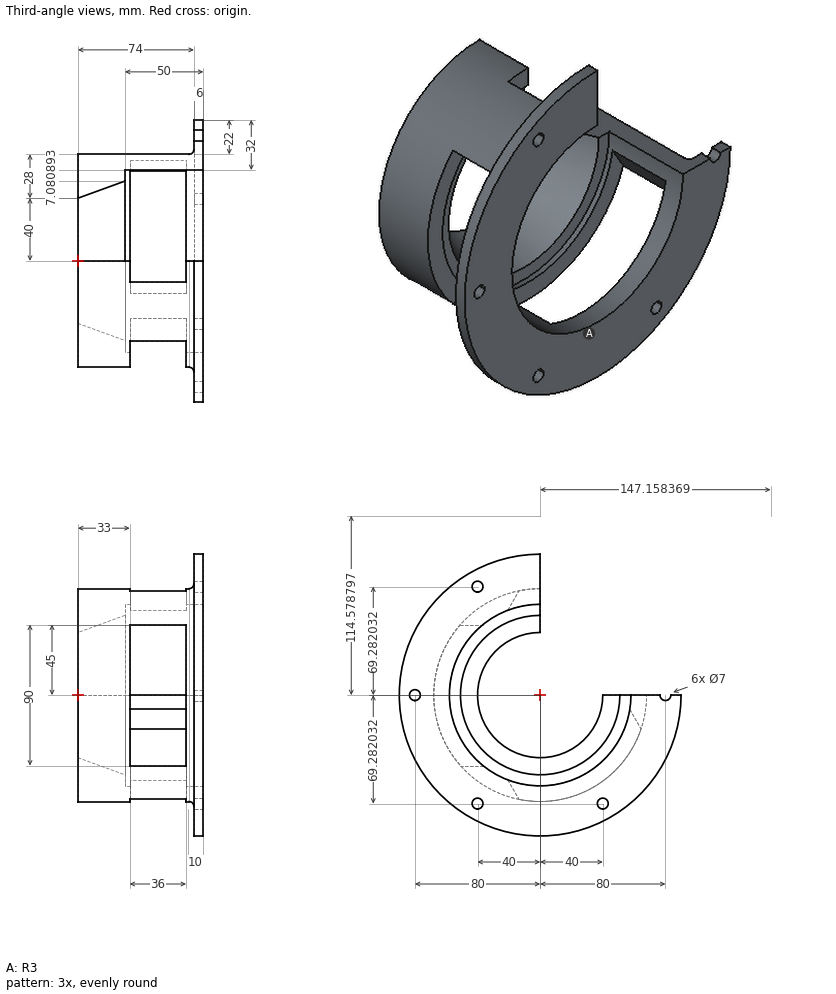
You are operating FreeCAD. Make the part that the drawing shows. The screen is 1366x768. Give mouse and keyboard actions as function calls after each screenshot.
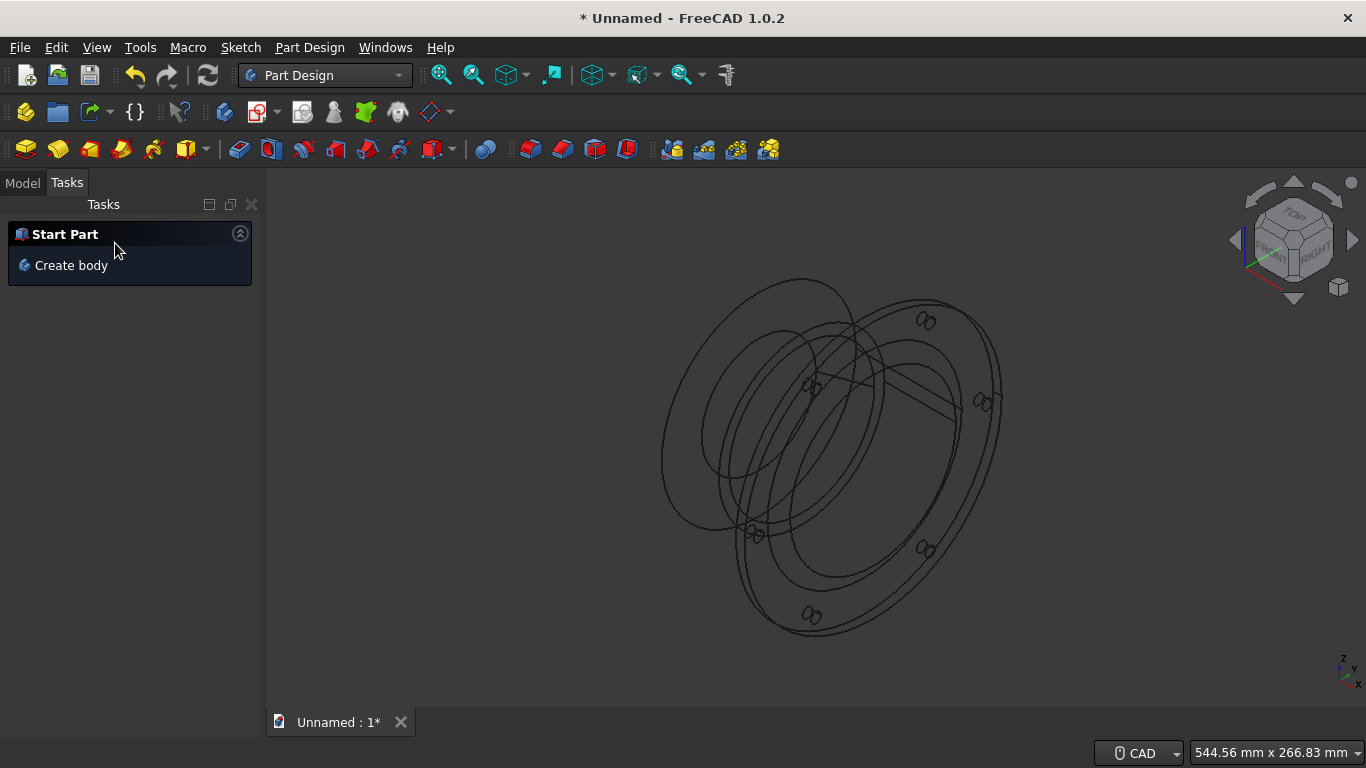
click(767, 521)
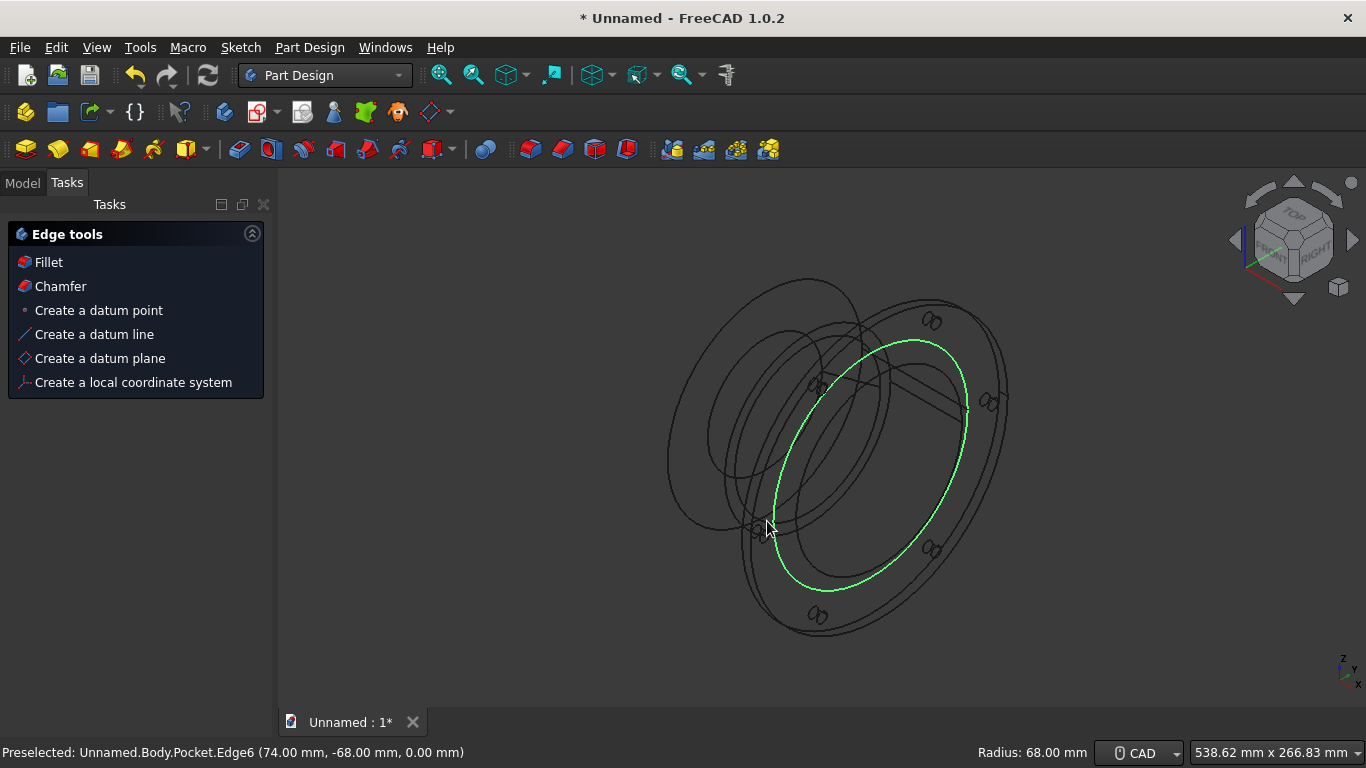
key(v)
key(1)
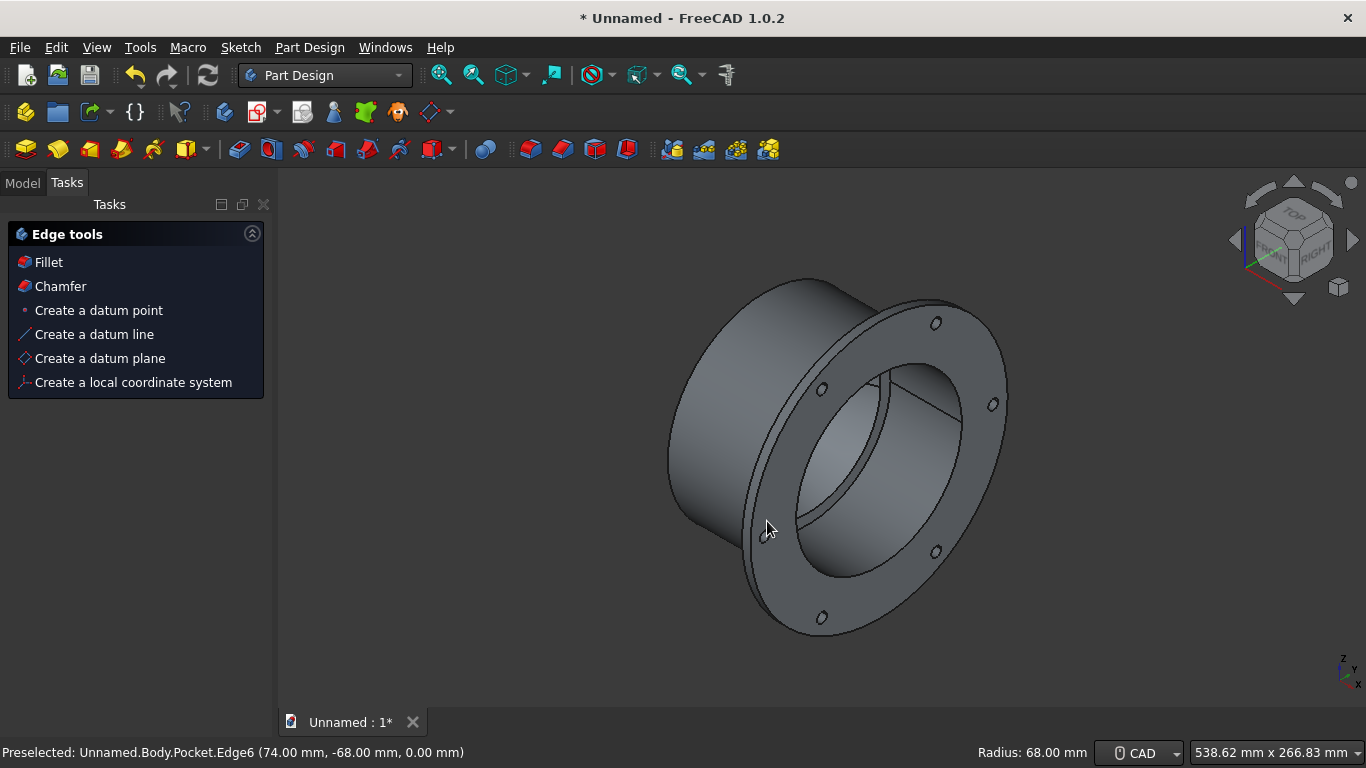
click(532, 150)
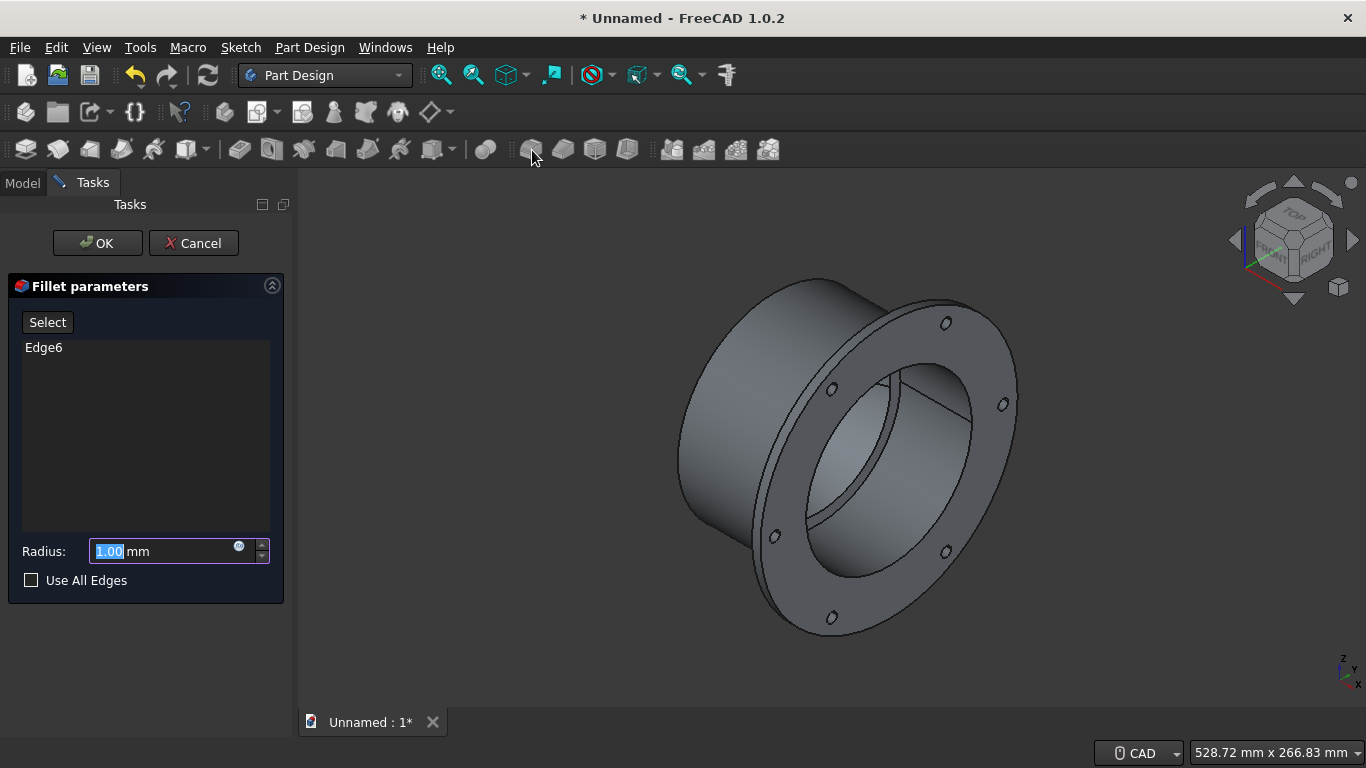
text(3)
key(Tab)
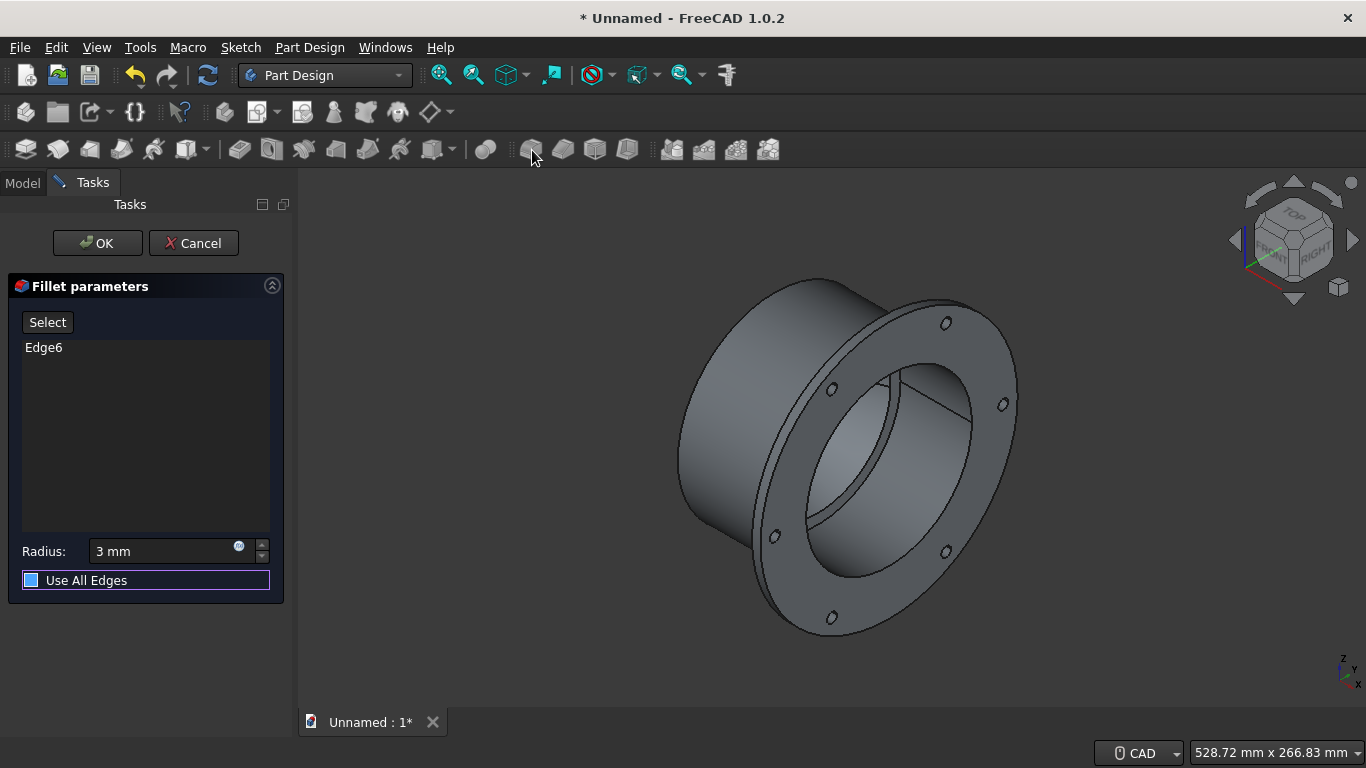
click(98, 243)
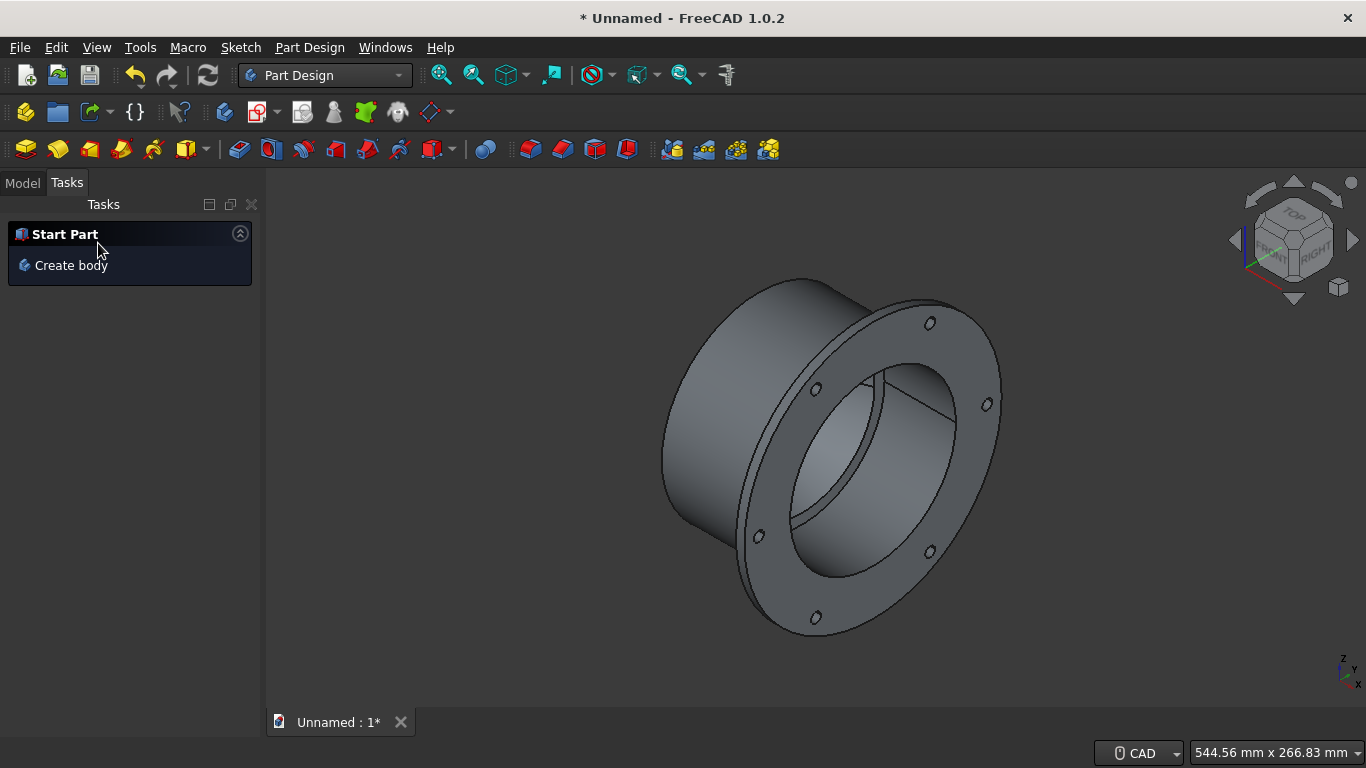
click(258, 112)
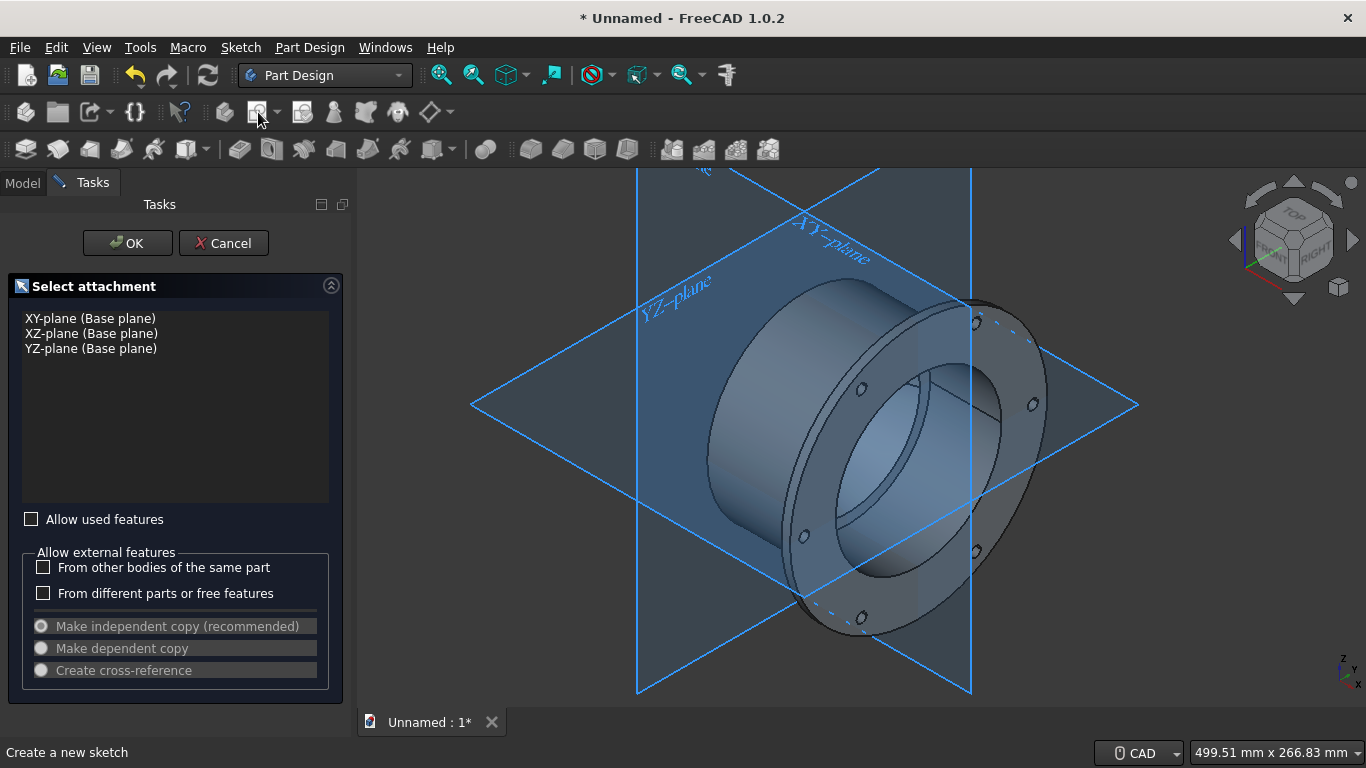
click(82, 334)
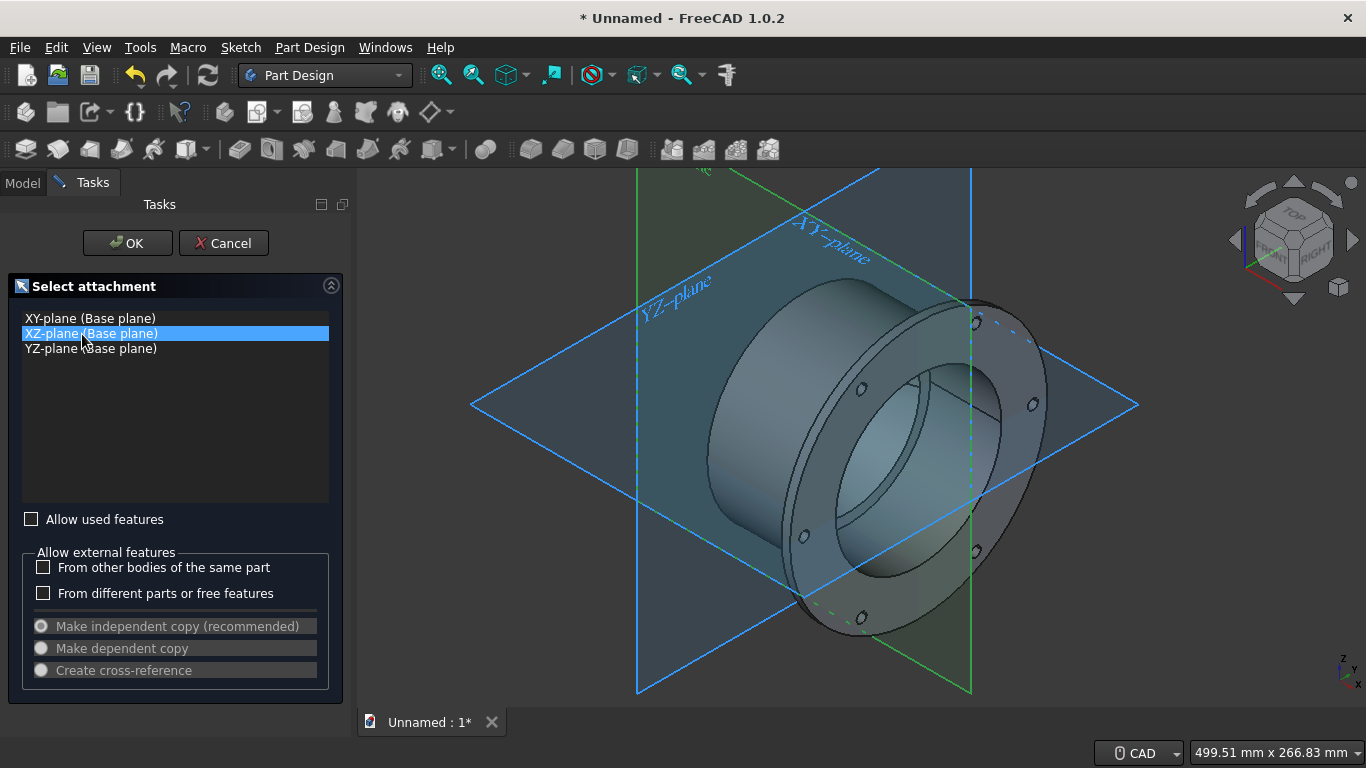
click(128, 243)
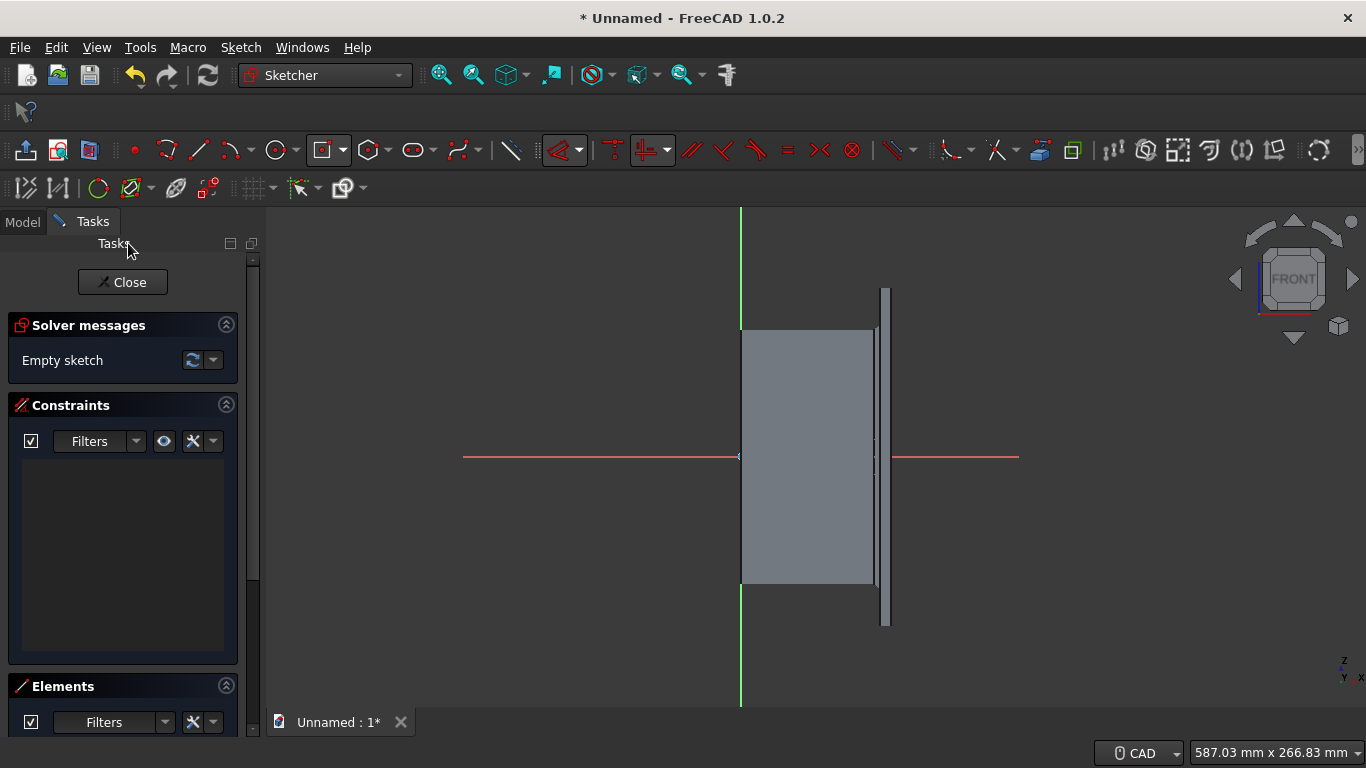
key(q)
key(s)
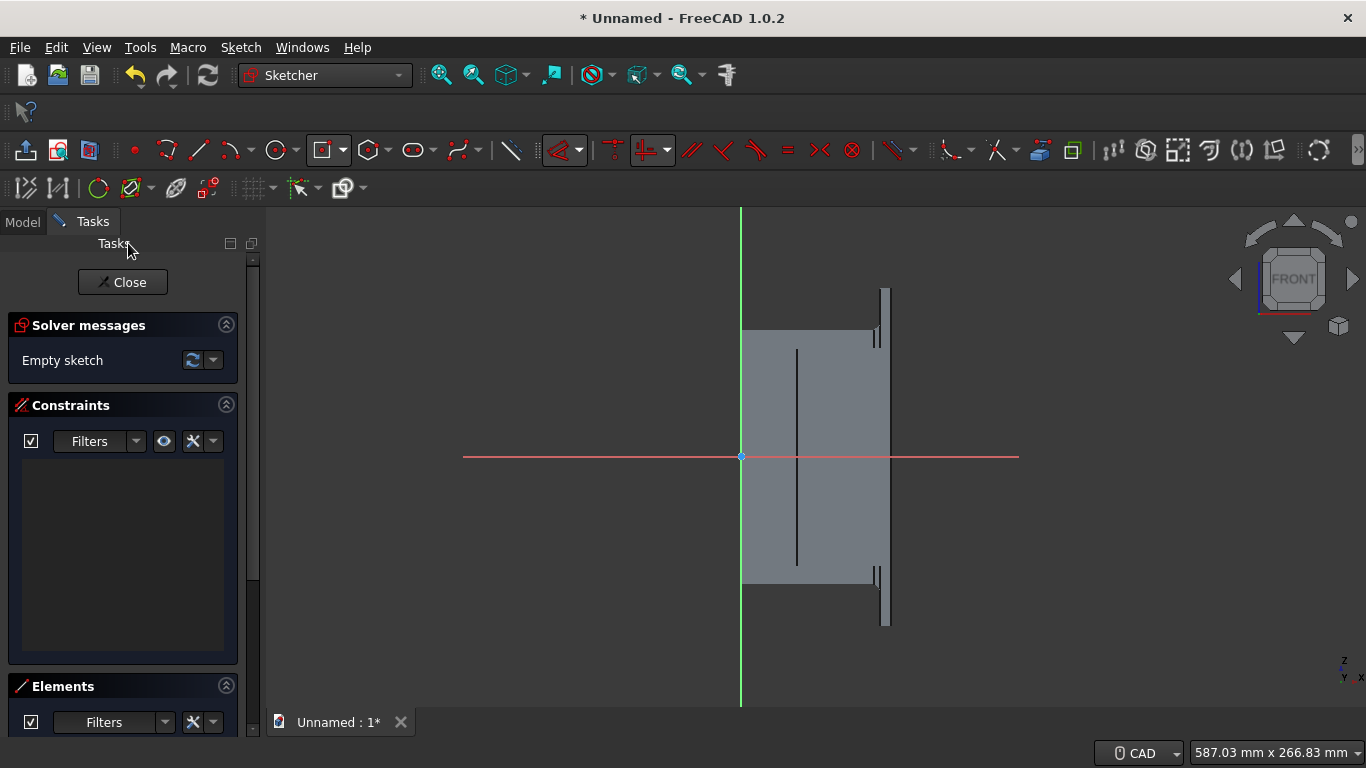
scroll(876, 457, up, 3)